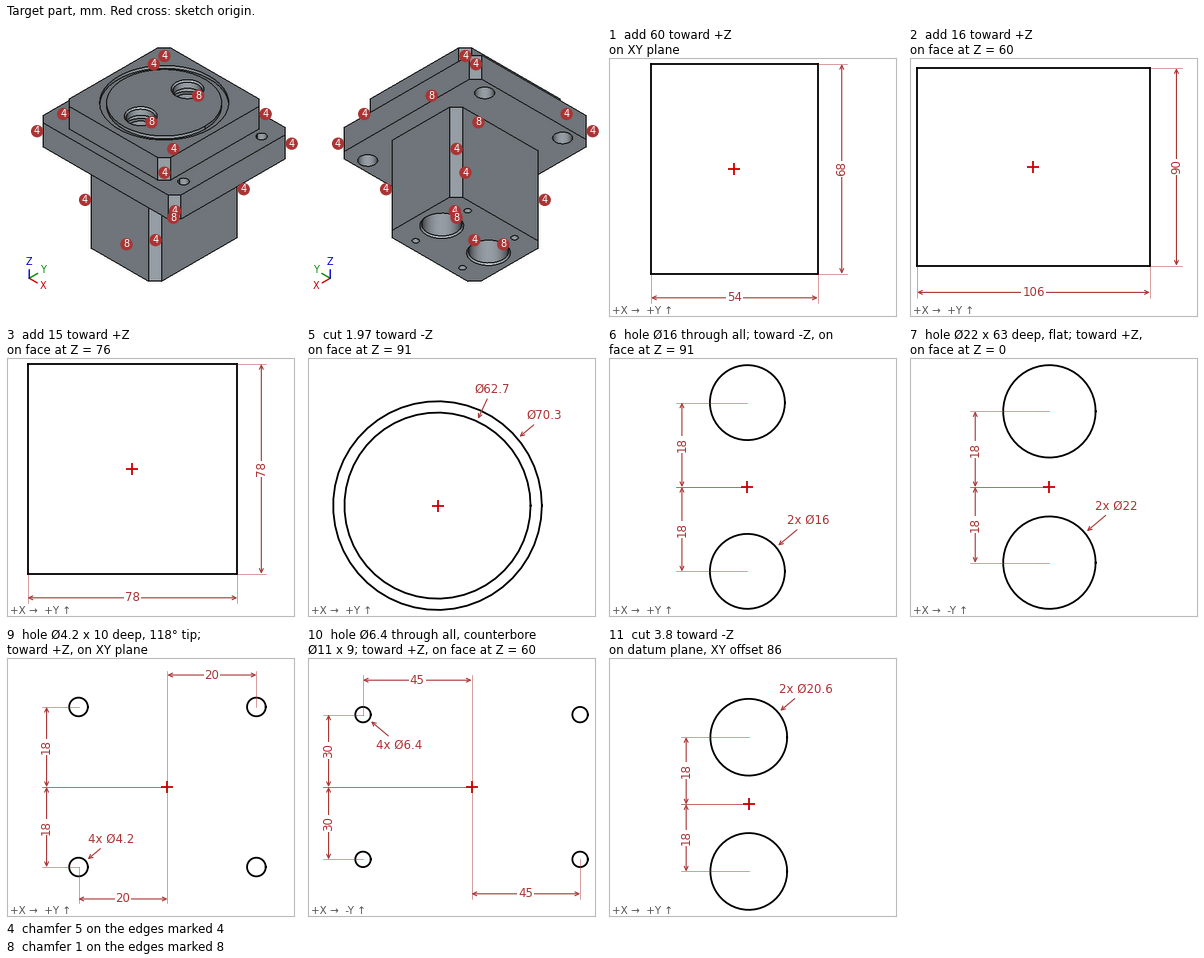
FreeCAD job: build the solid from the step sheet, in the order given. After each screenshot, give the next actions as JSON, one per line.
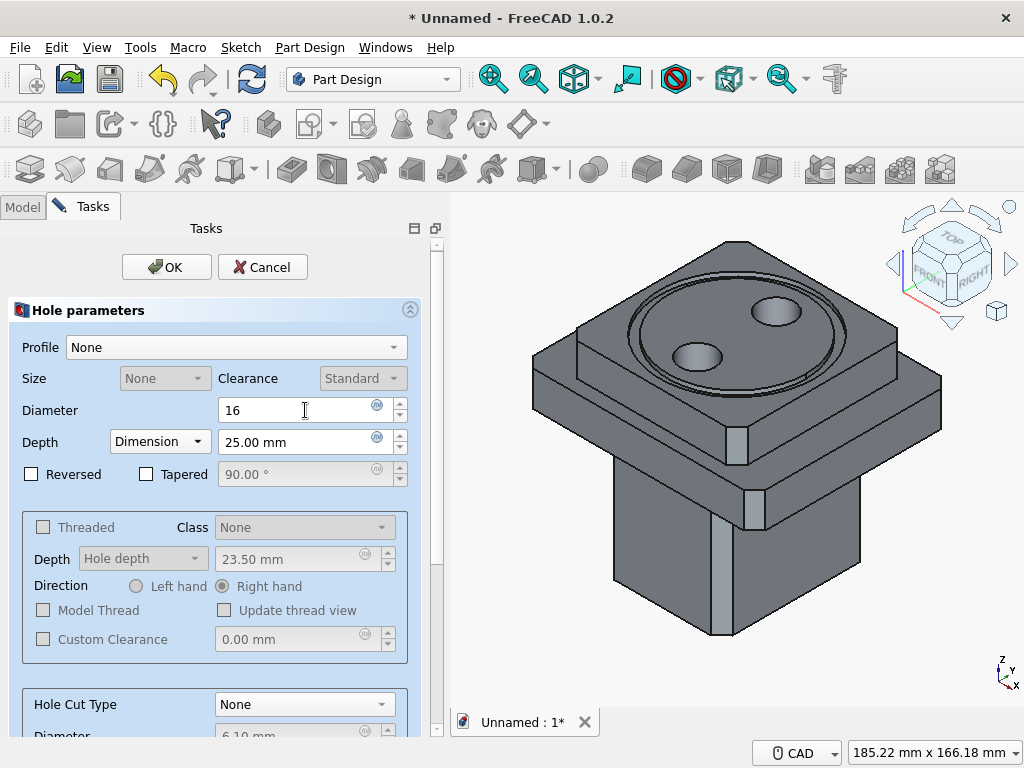
{"action": "left_click", "coordinate": [161, 442]}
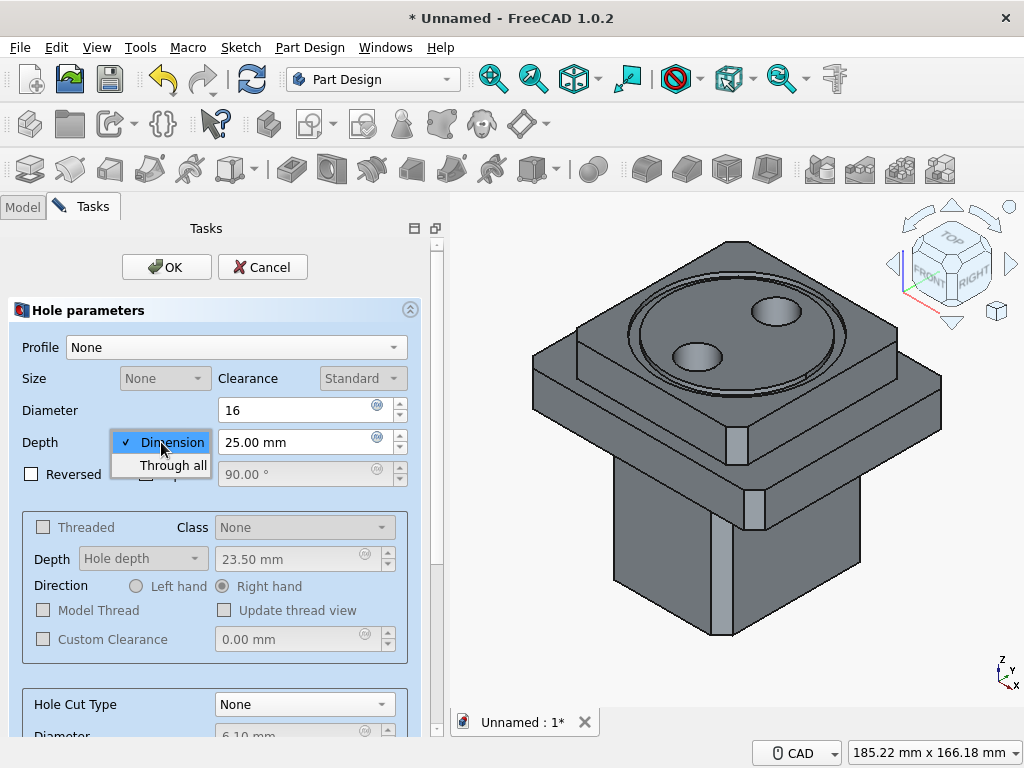
{"action": "left_click", "coordinate": [160, 466]}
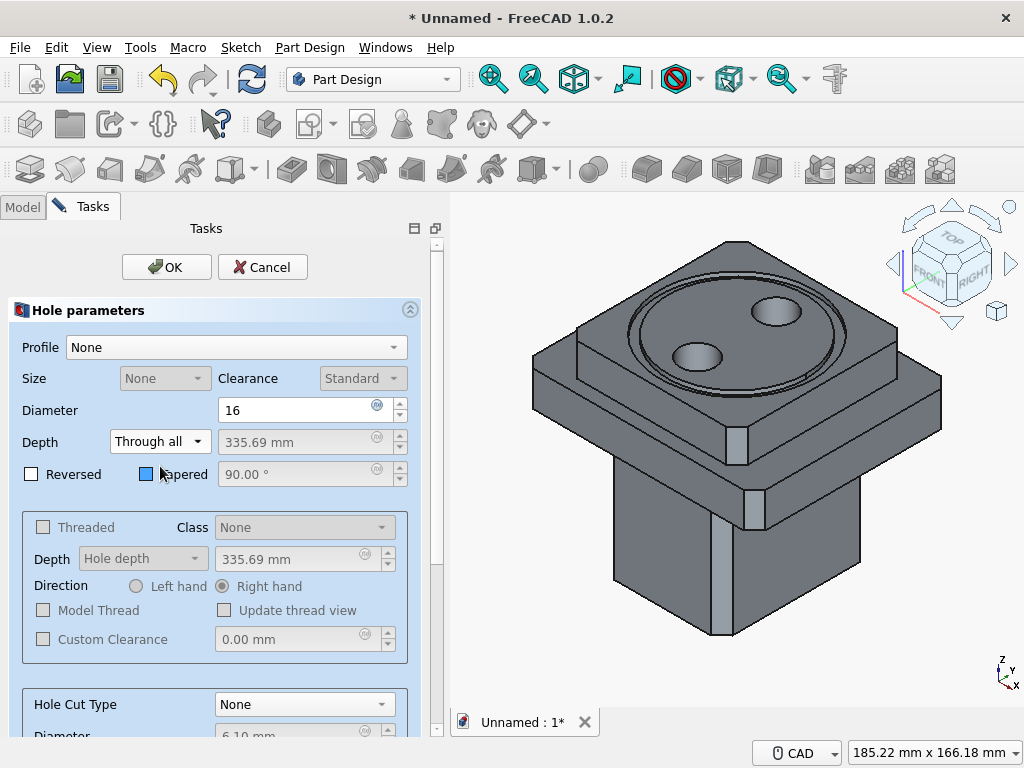
{"action": "left_click", "coordinate": [167, 267]}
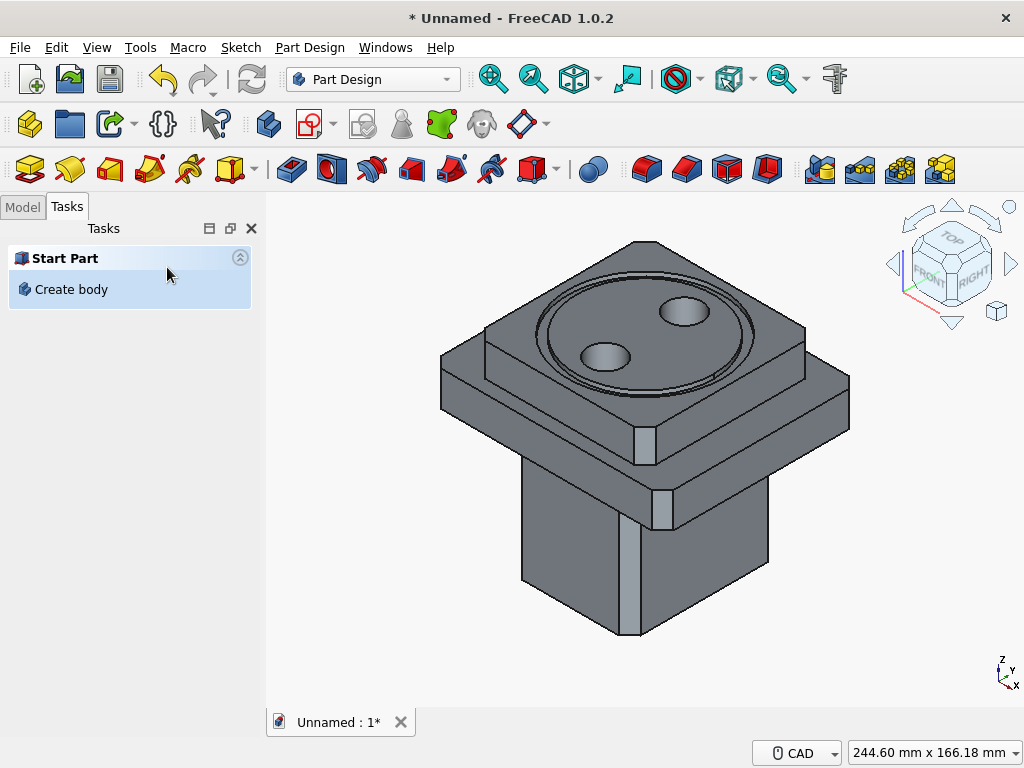
{"action": "key", "text": "5"}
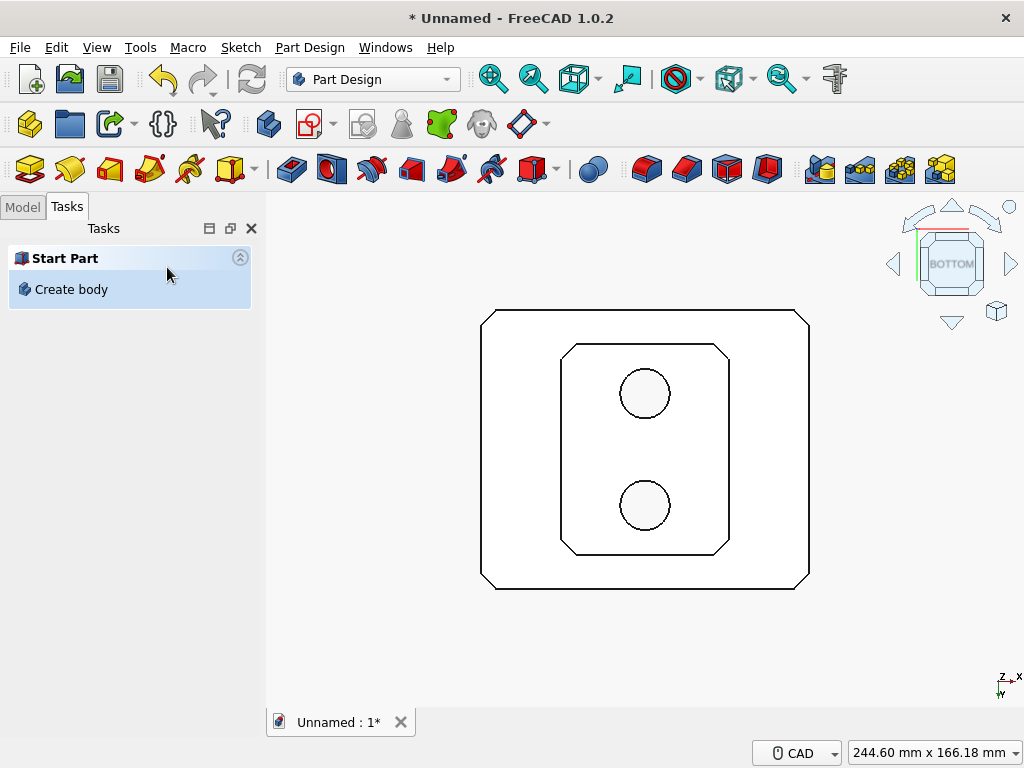
{"action": "left_click", "coordinate": [621, 449]}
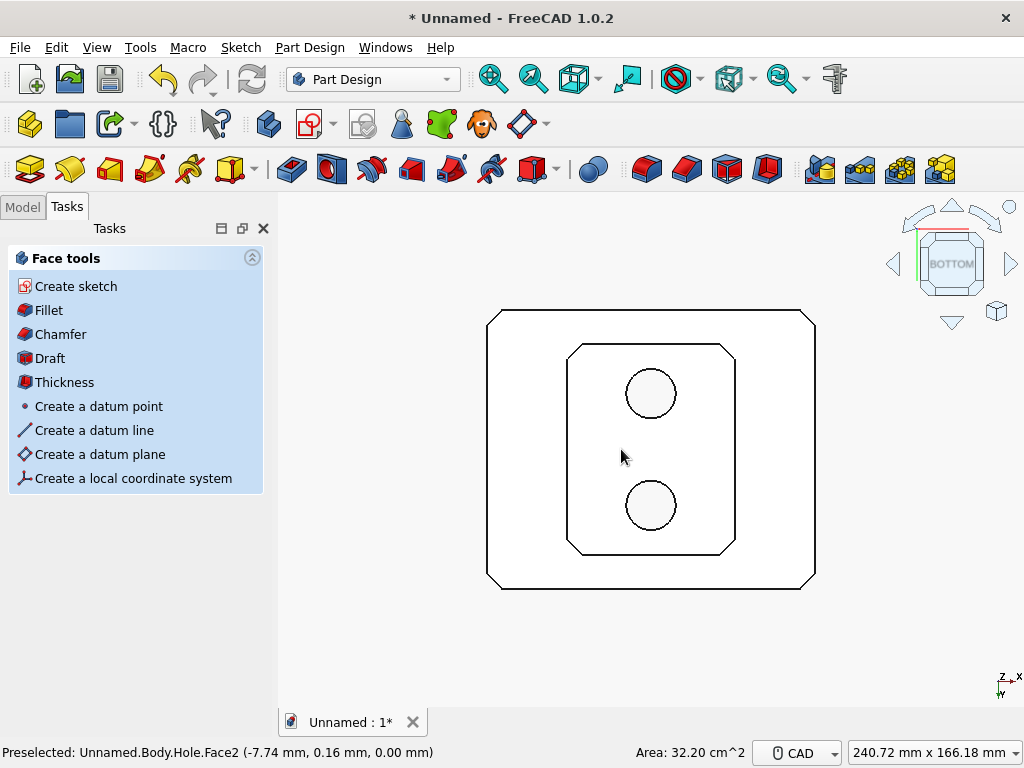
{"action": "left_click", "coordinate": [310, 124]}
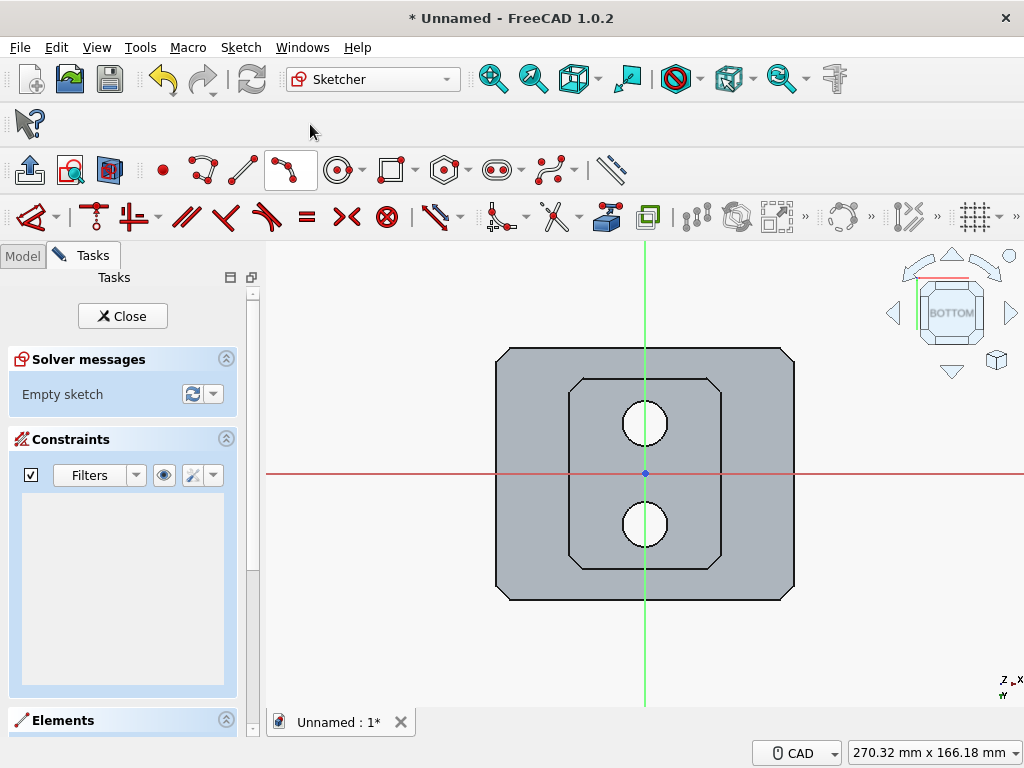
{"action": "scroll", "coordinate": [728, 474], "scroll_direction": "up", "scroll_amount": 3}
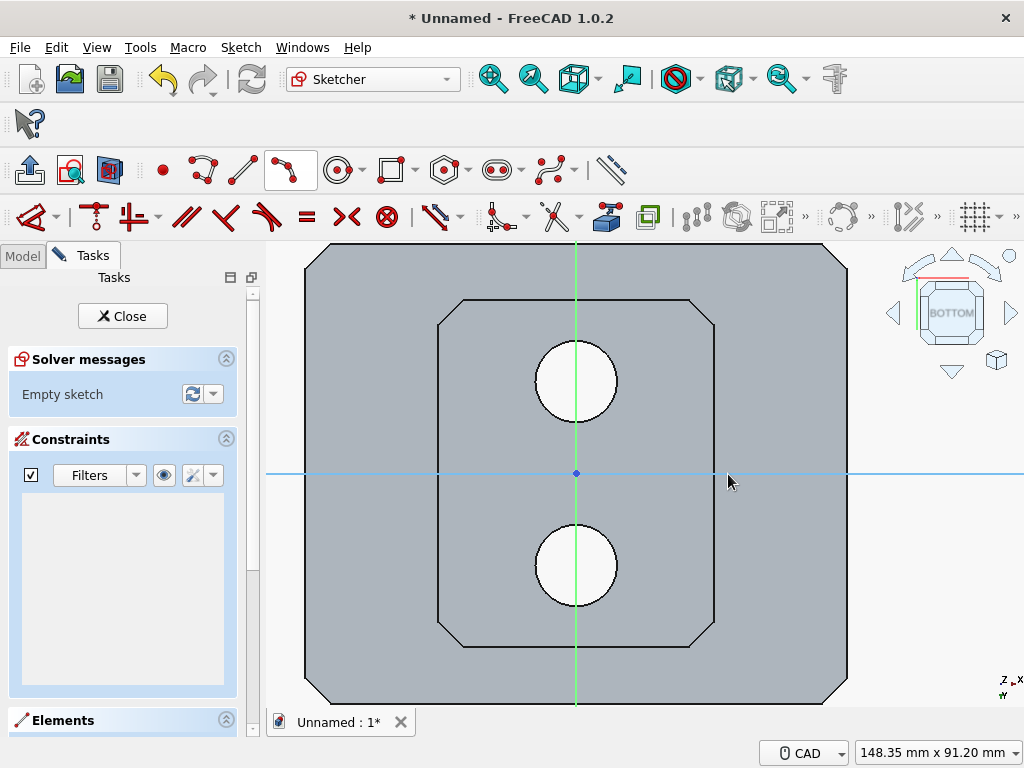
{"action": "left_click", "coordinate": [338, 170]}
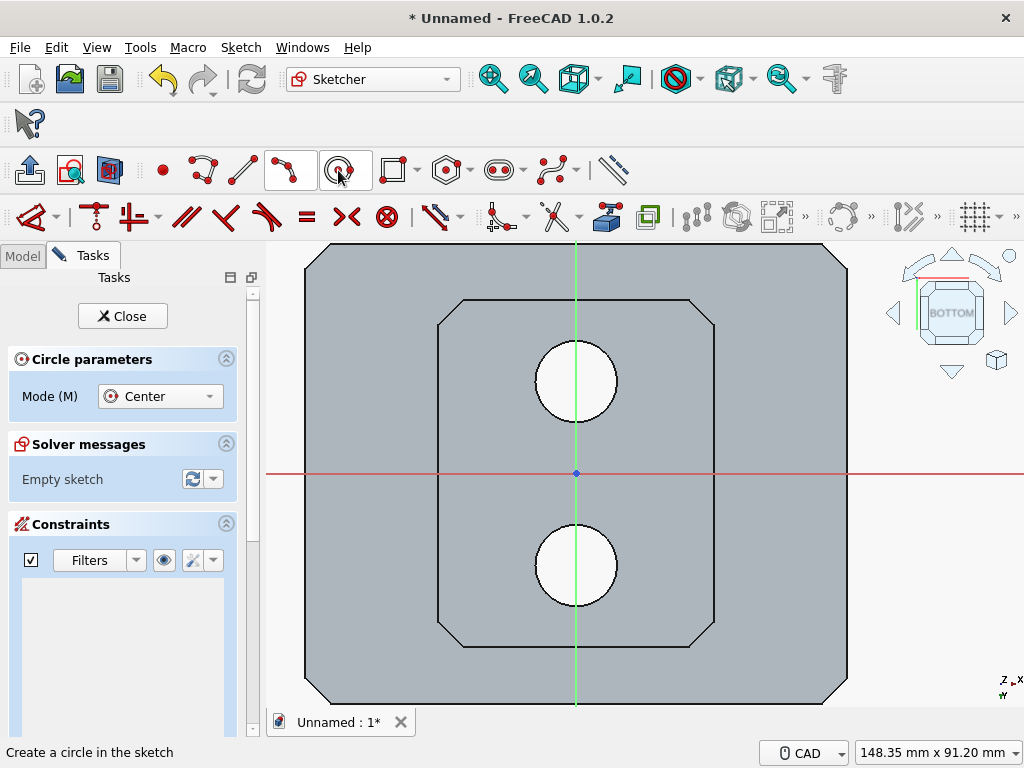
{"action": "left_click", "coordinate": [576, 566]}
{"action": "mouse_move", "coordinate": [616, 526]}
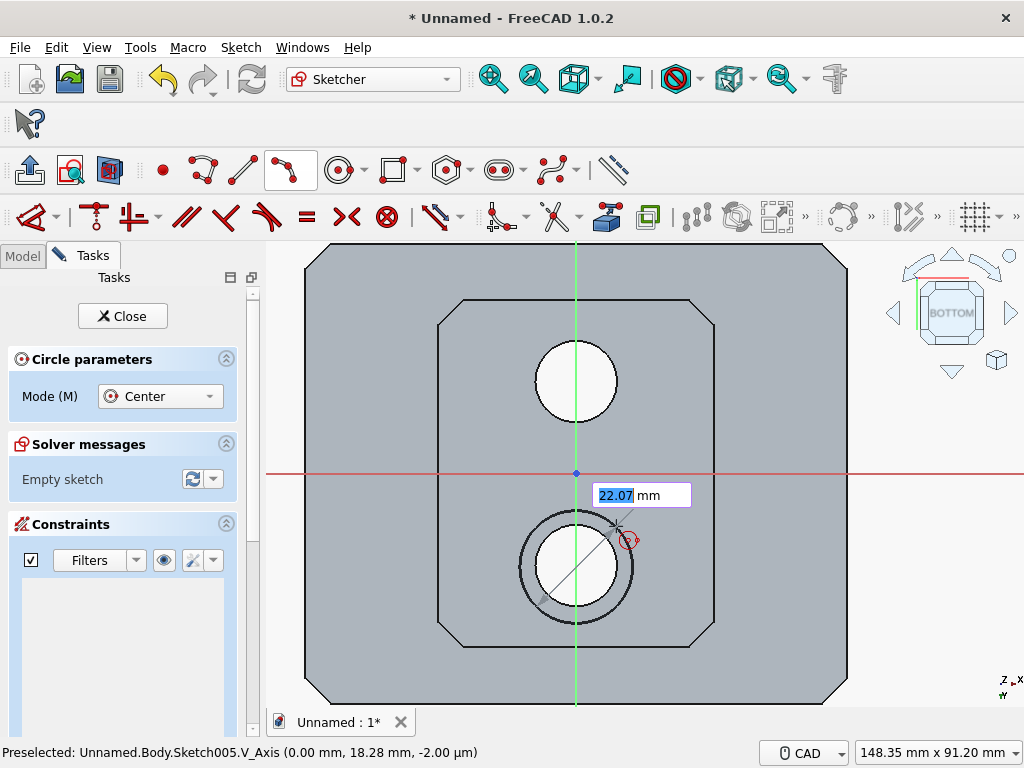
{"action": "type", "text": "22"}
{"action": "key", "text": "Return"}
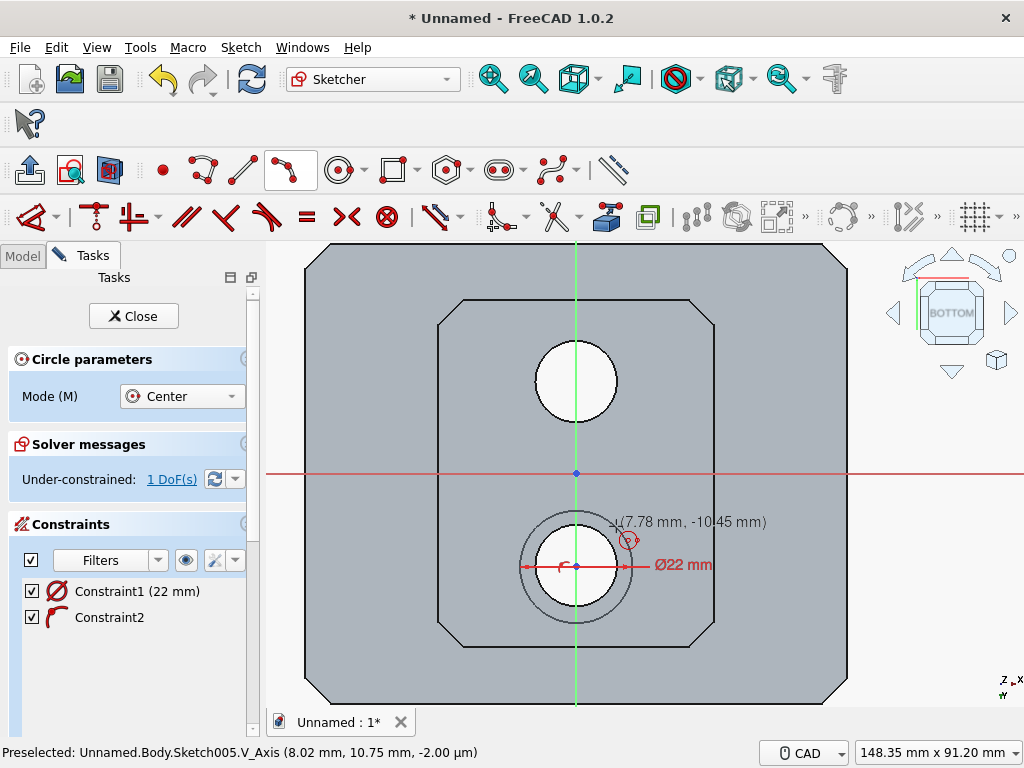
{"action": "left_click", "coordinate": [576, 382]}
{"action": "mouse_move", "coordinate": [616, 342]}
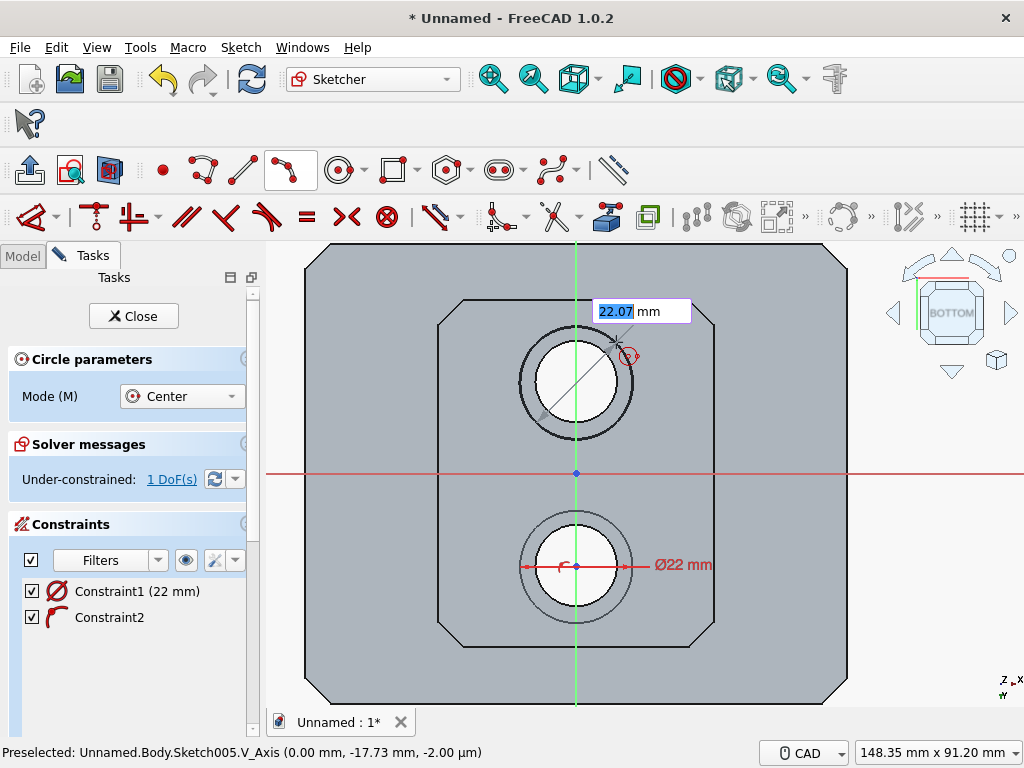
{"action": "type", "text": "22"}
{"action": "key", "text": "Return"}
{"action": "key", "text": "Escape"}